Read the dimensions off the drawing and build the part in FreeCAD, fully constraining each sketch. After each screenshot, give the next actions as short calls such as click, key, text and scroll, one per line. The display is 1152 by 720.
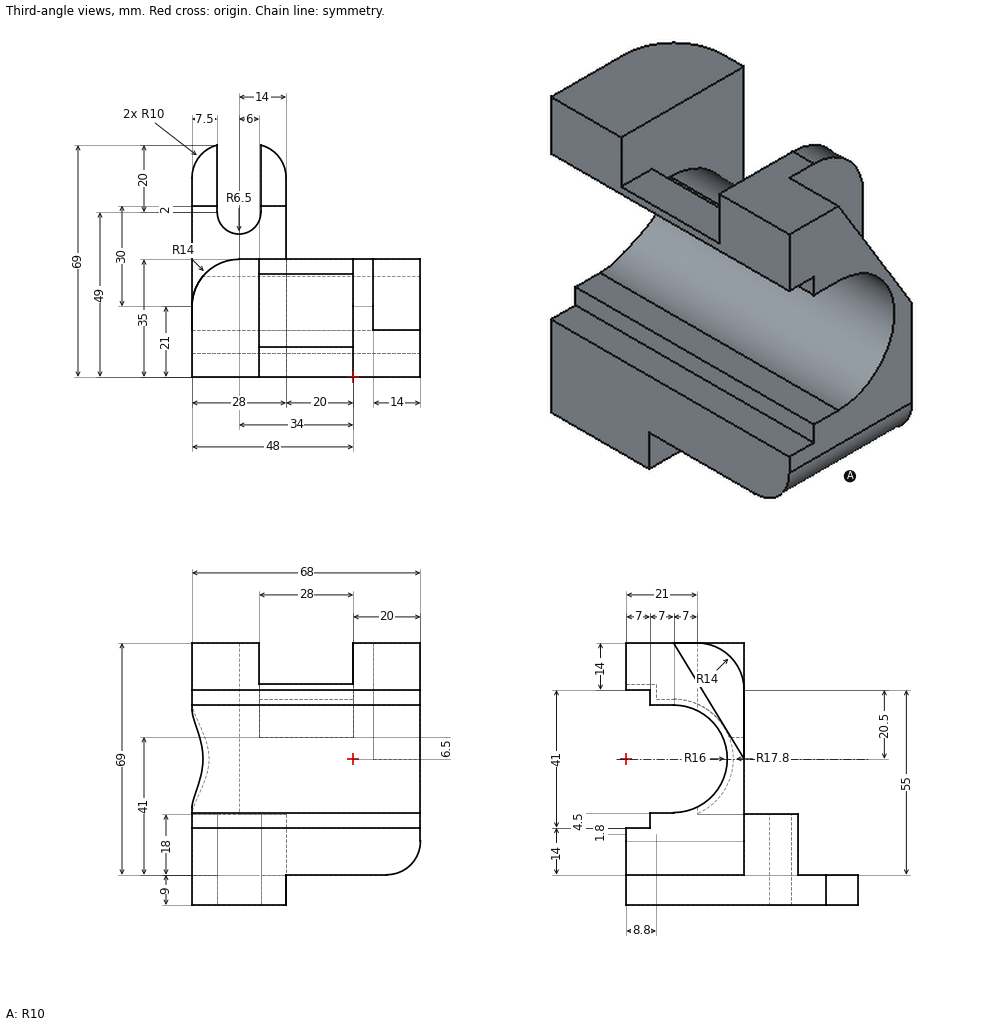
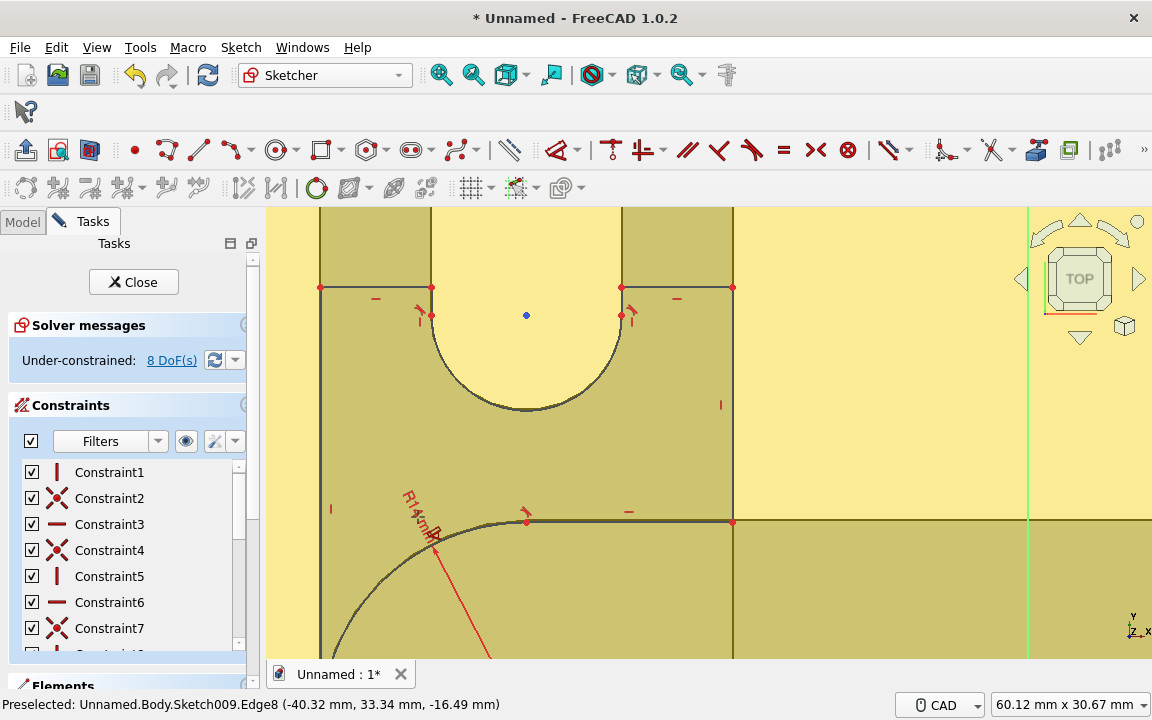
click(471, 393)
click(452, 419)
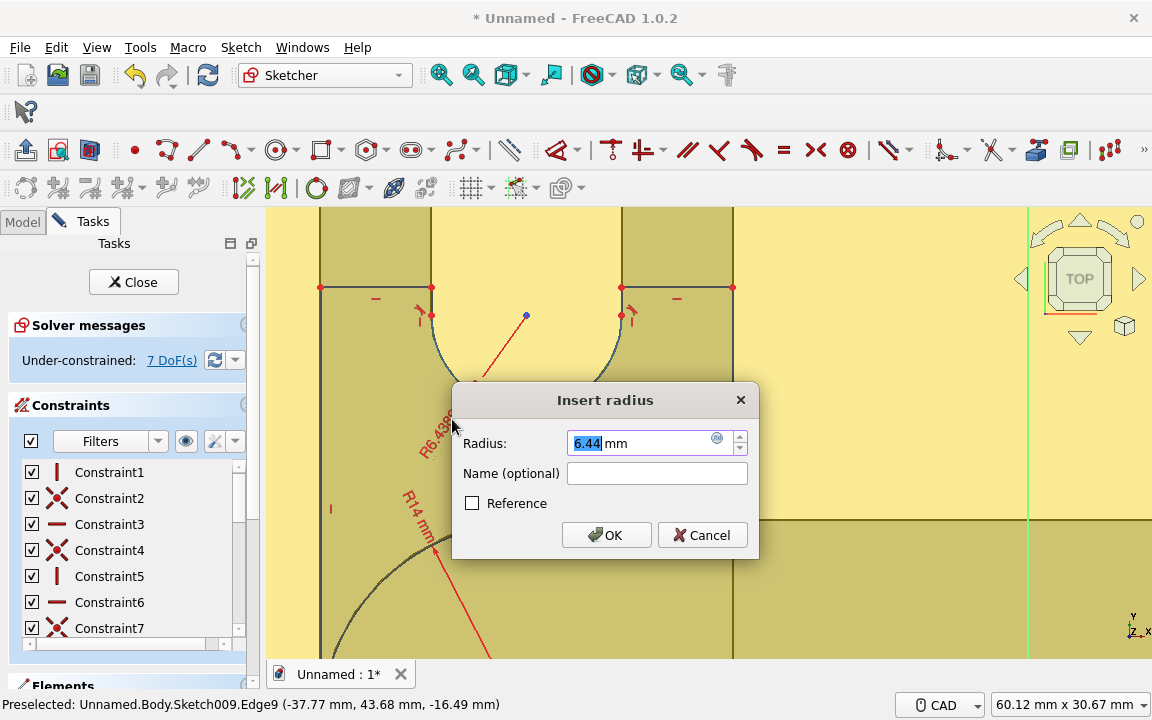
text(6.5)
key(Return)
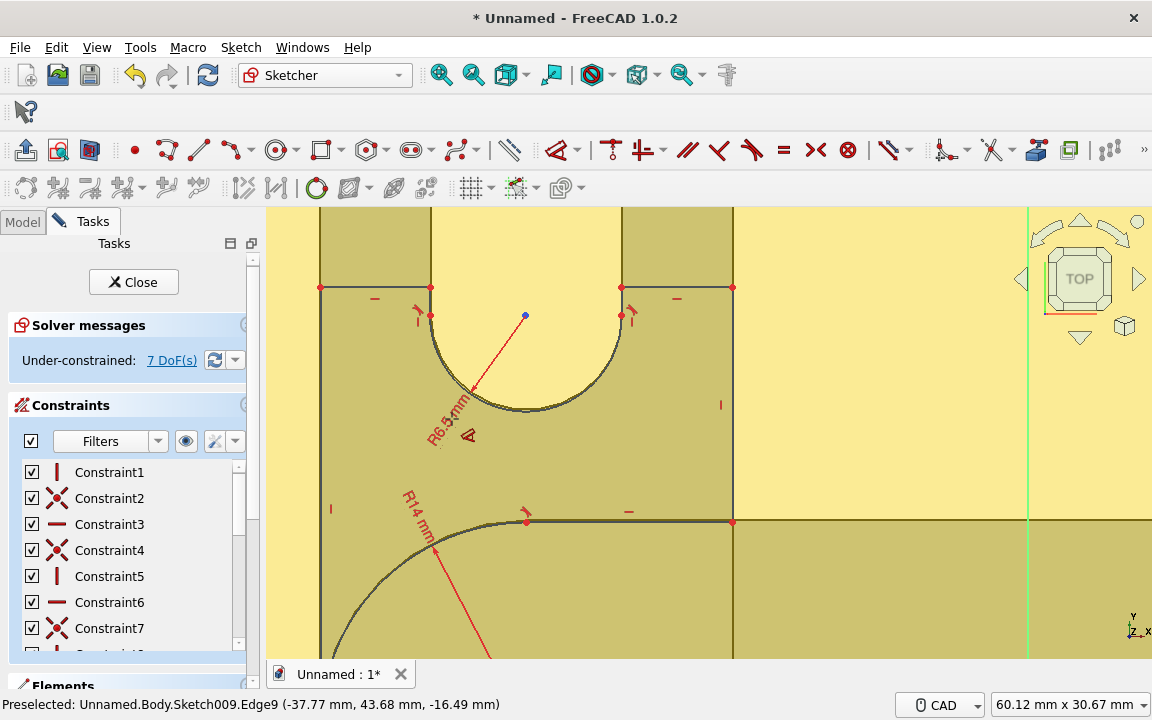
scroll(430, 304, up, 2)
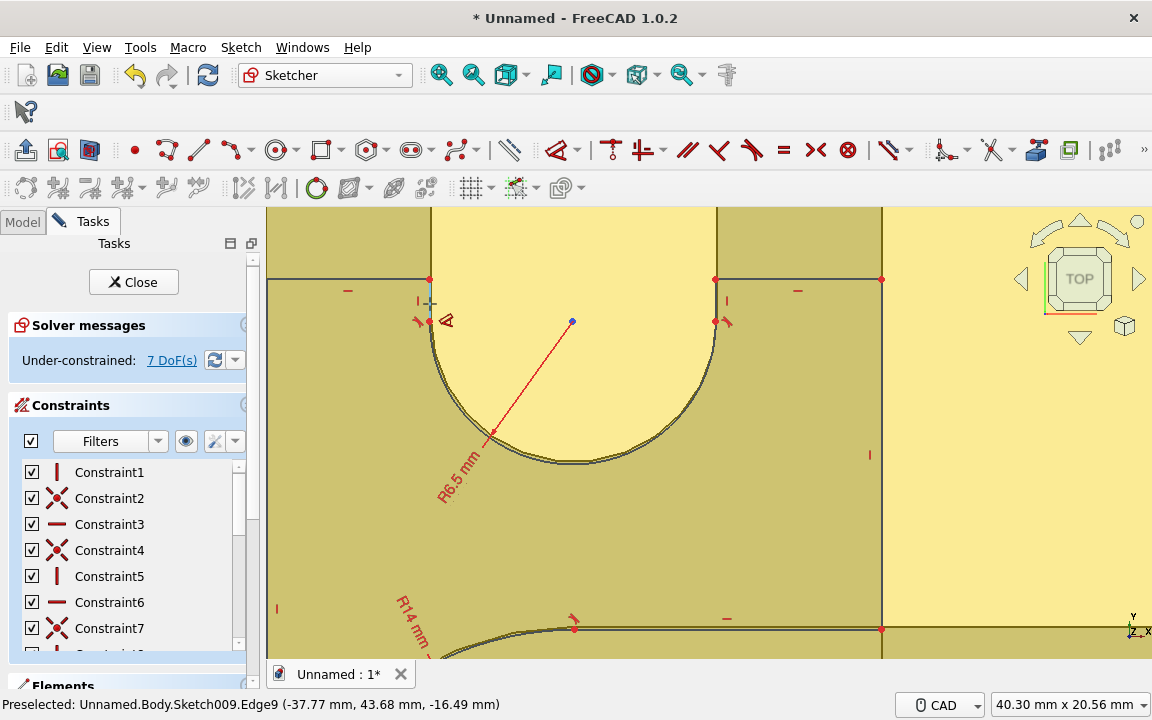
click(430, 305)
click(396, 300)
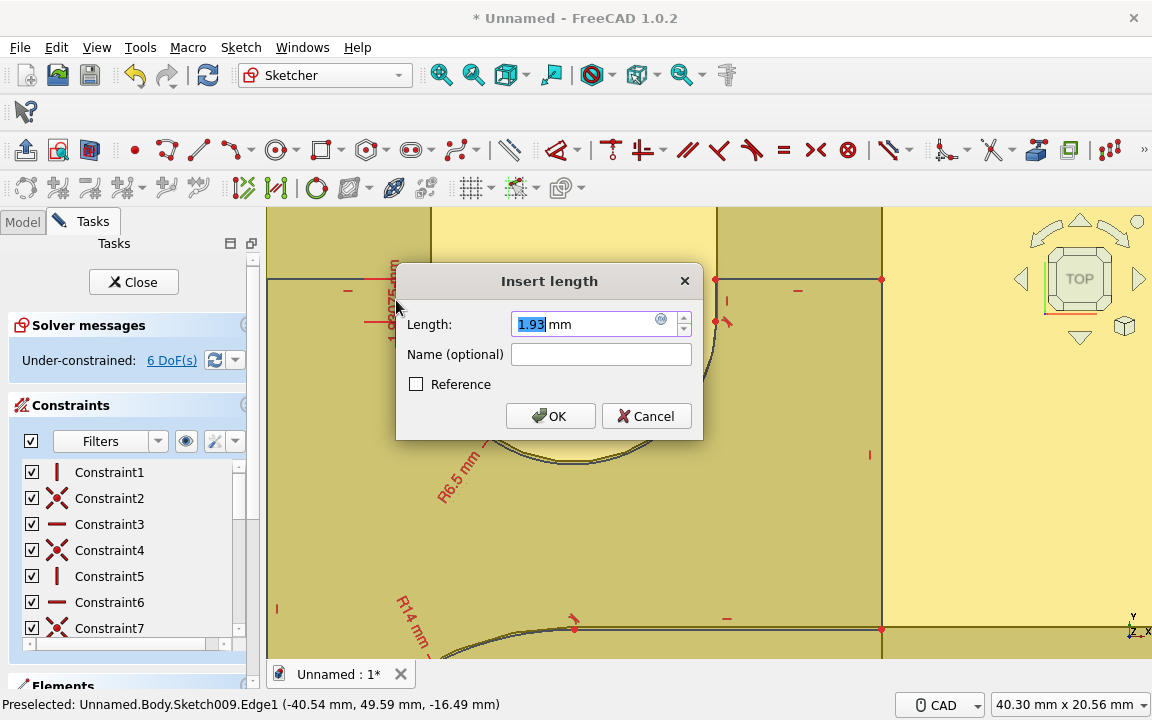
text(2)
key(Return)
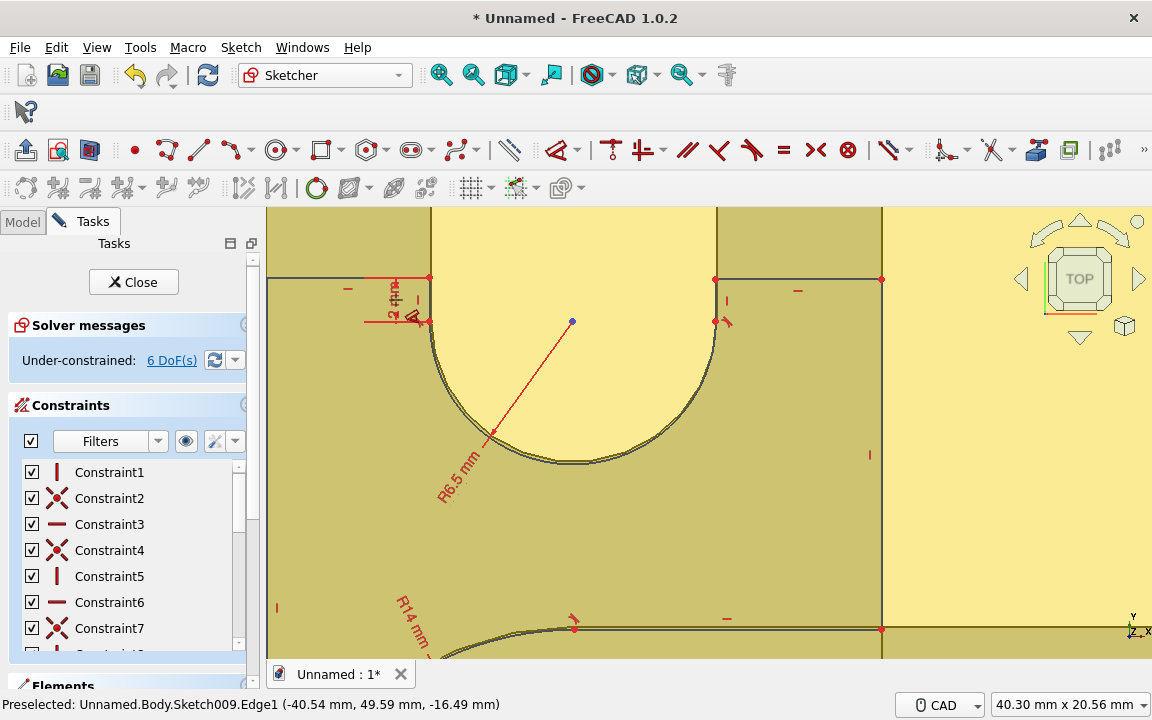
click(716, 292)
click(682, 300)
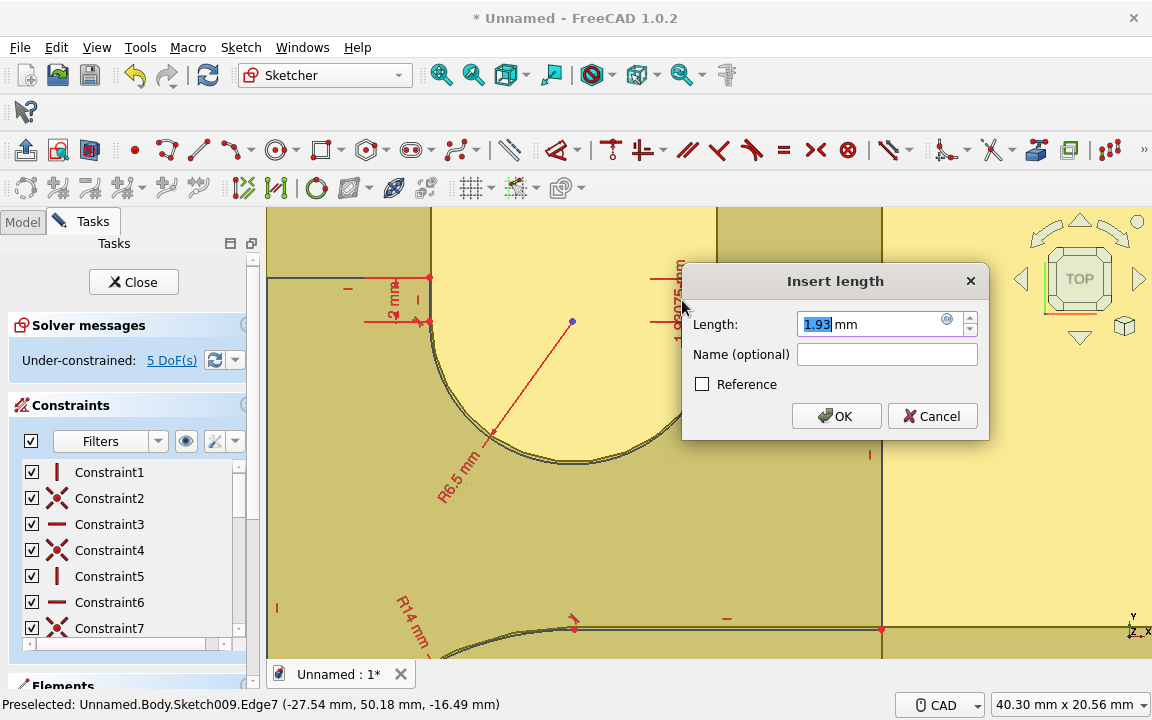
text(2)
key(Return)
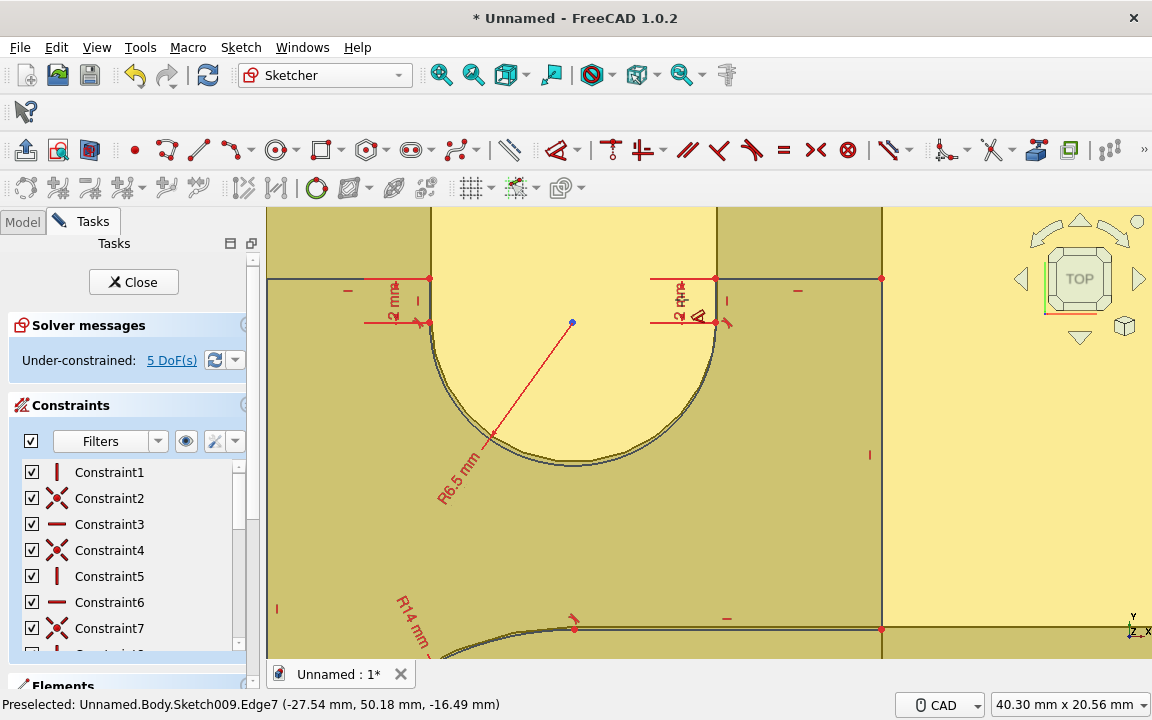
scroll(590, 301, down, 7)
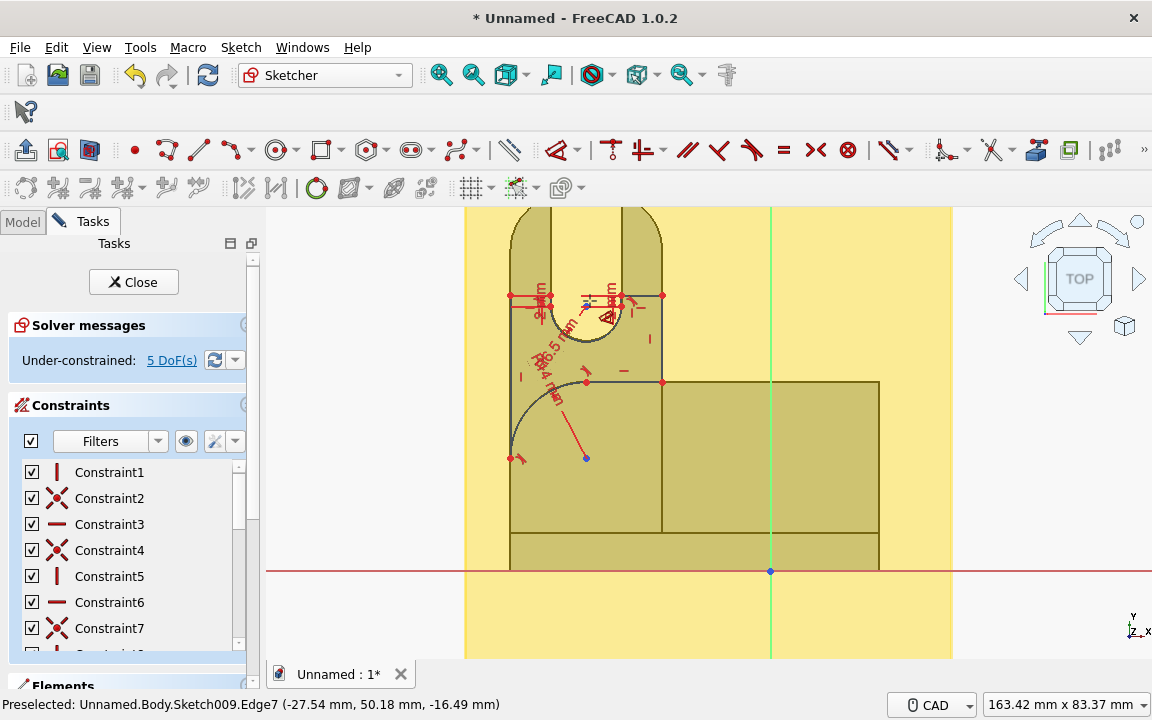
click(511, 344)
click(477, 377)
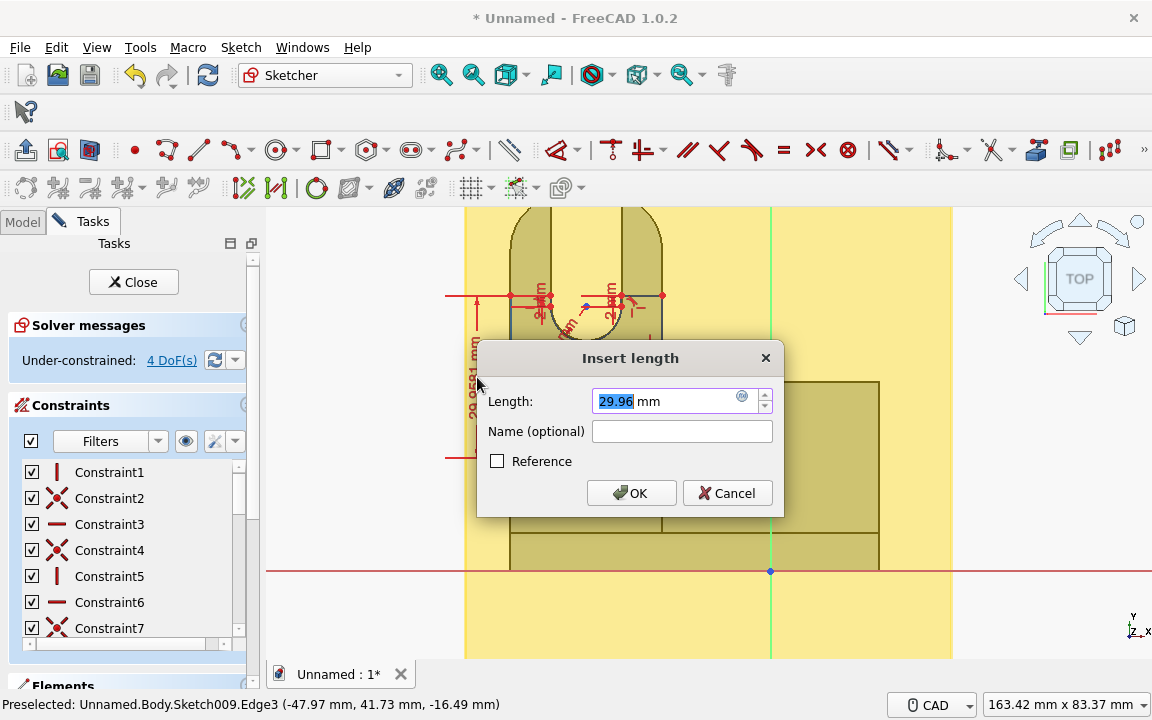
text(30)
key(Return)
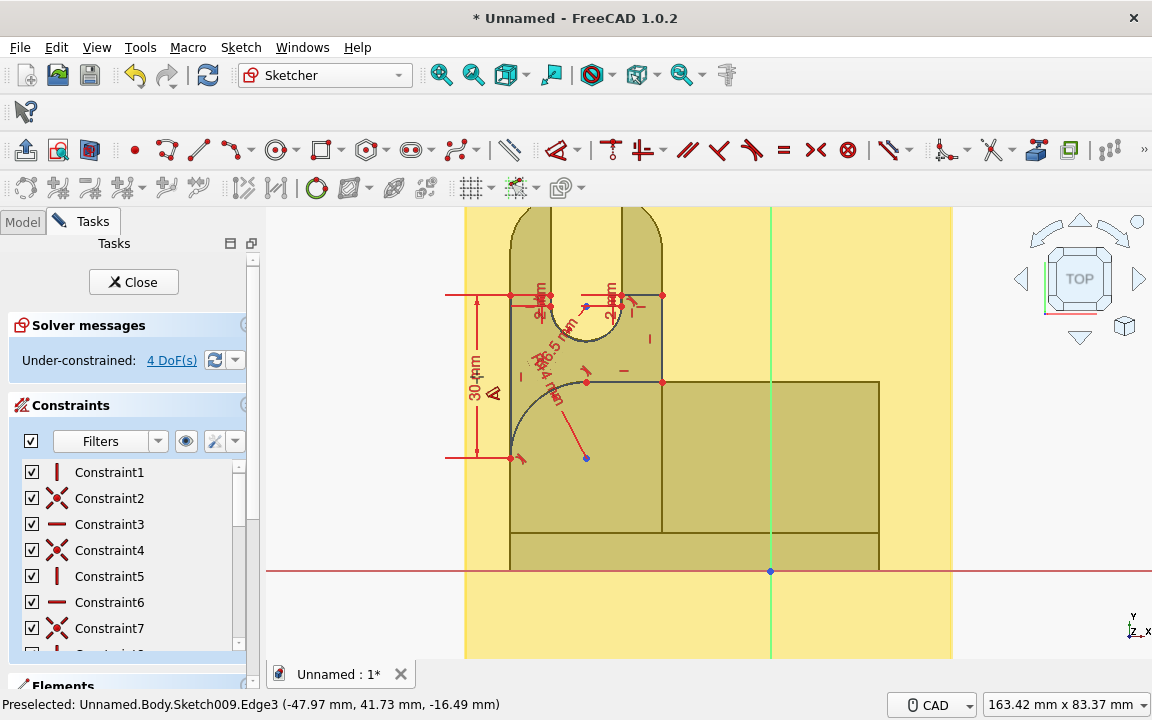
click(609, 382)
click(642, 348)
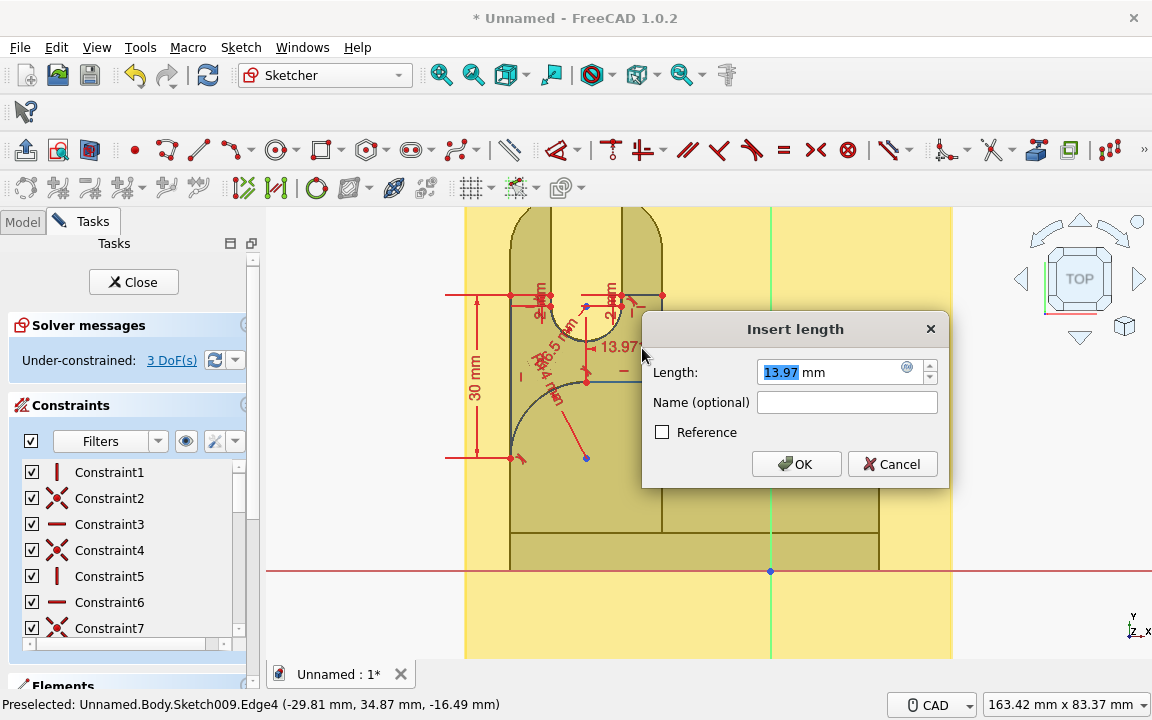
text(14)
key(Return)